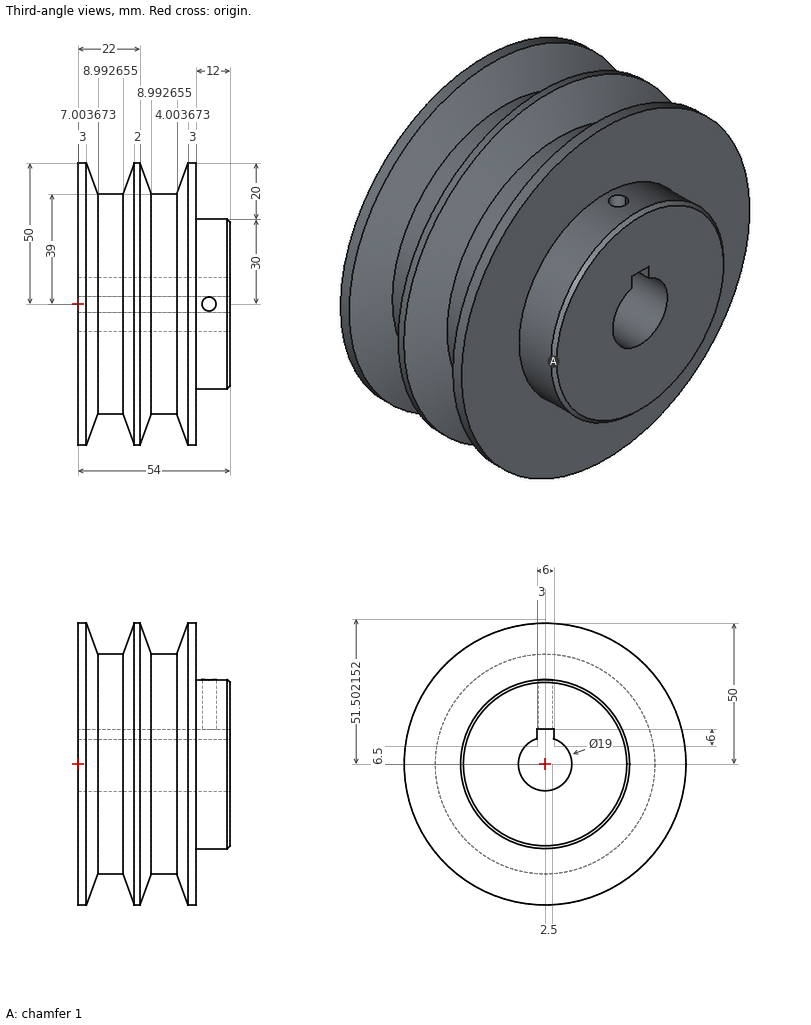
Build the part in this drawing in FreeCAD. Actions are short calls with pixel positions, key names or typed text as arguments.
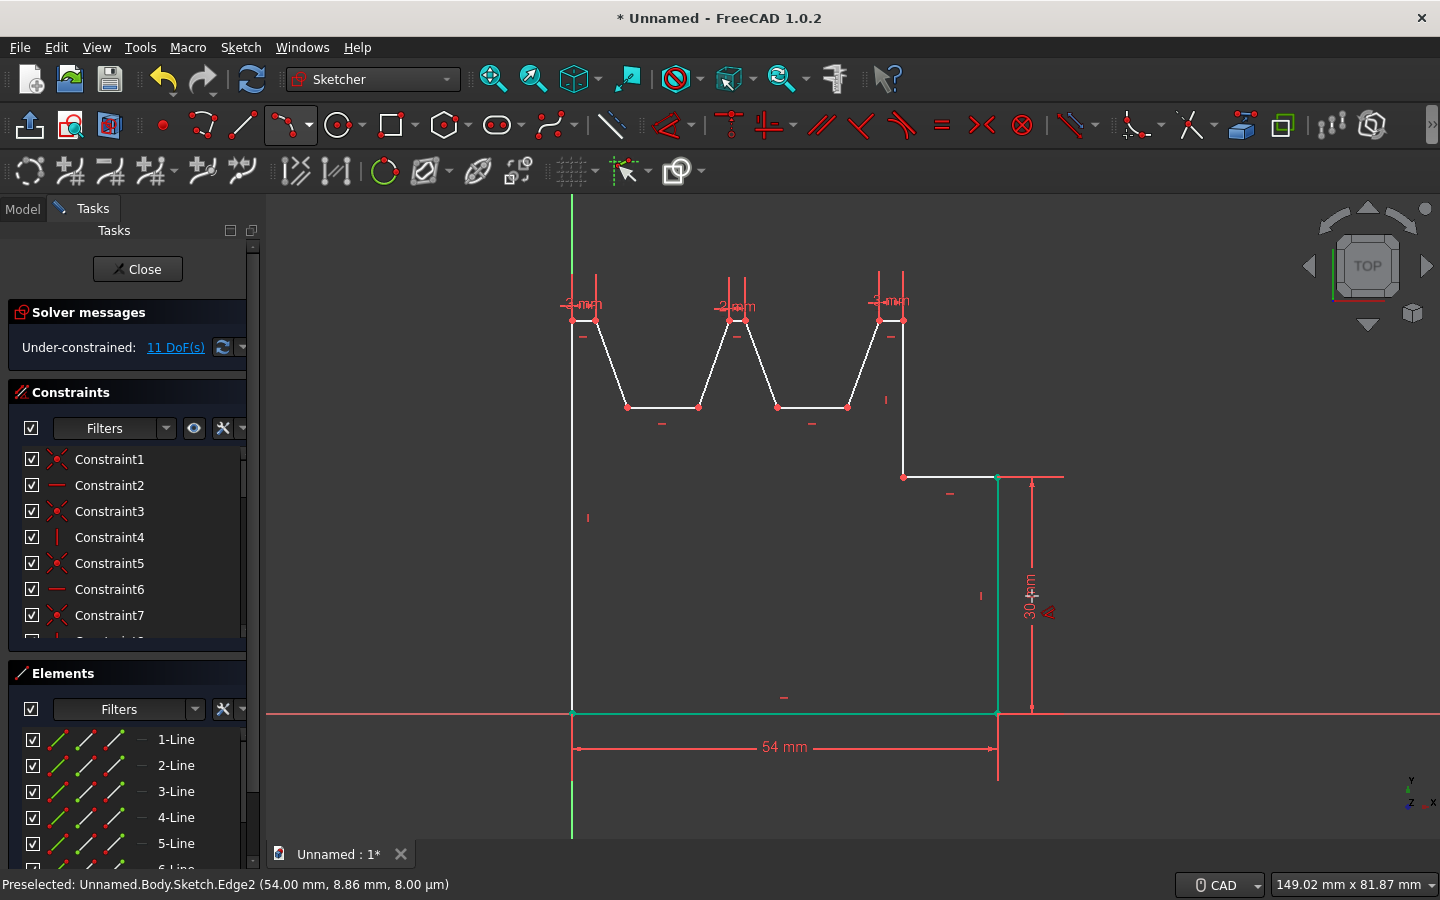
click(969, 477)
click(950, 443)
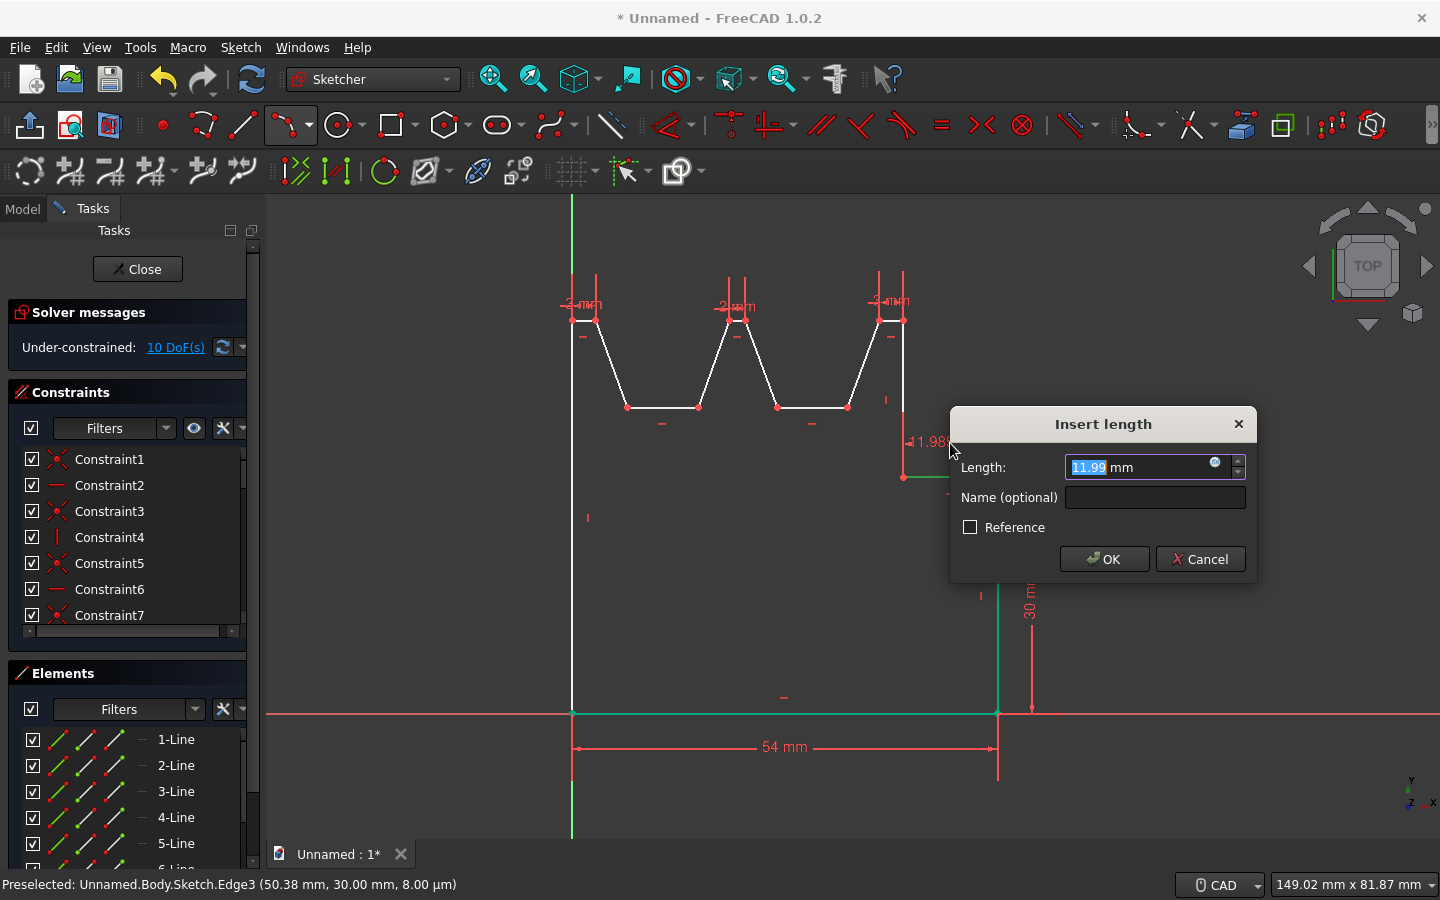
text(12)
key(Return)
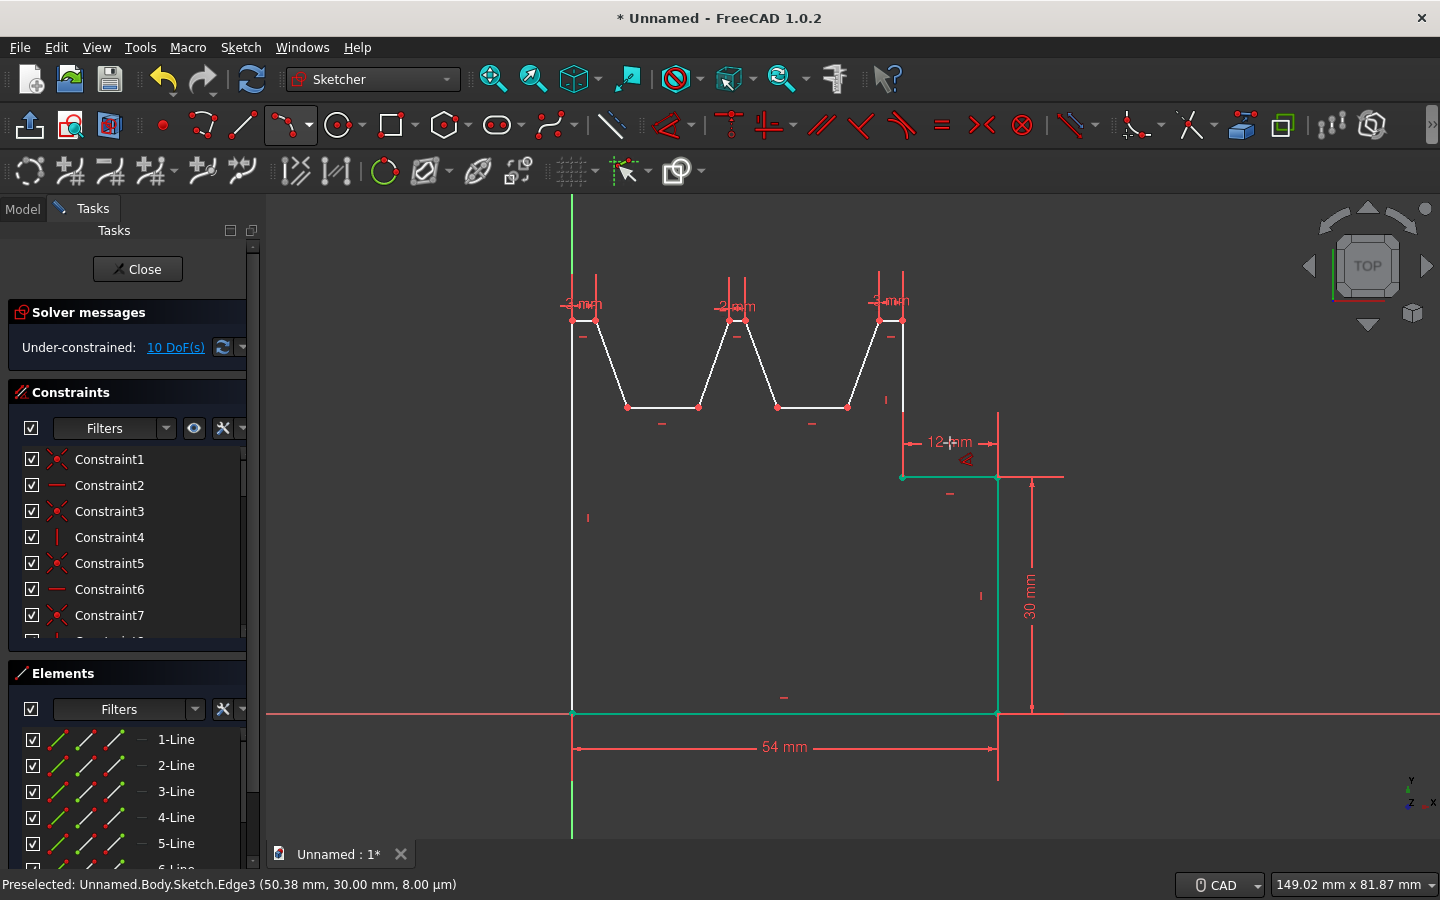
click(903, 430)
click(937, 399)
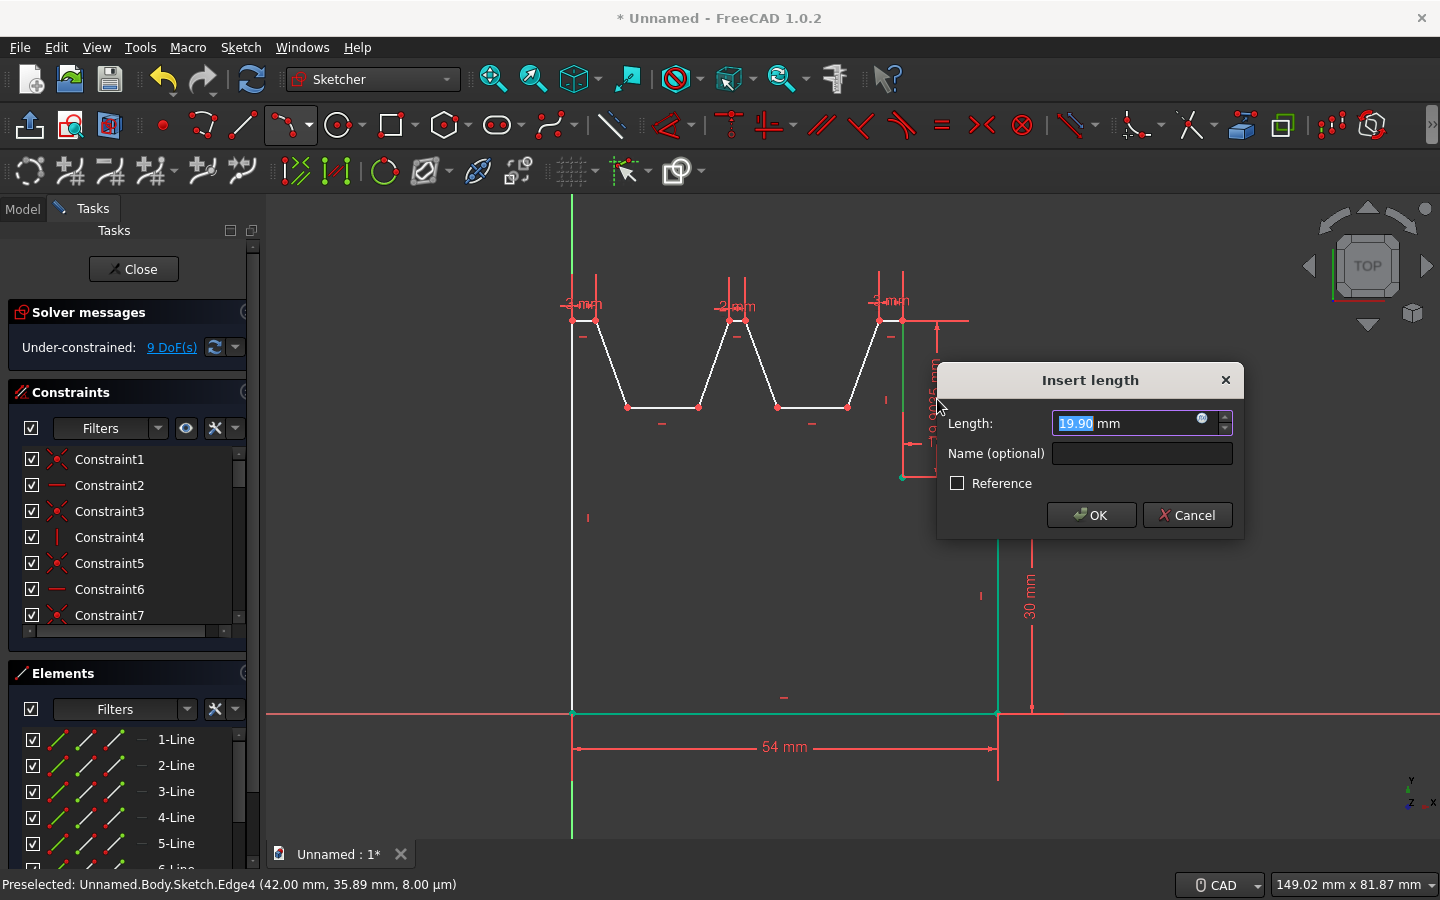
text(20)
key(Return)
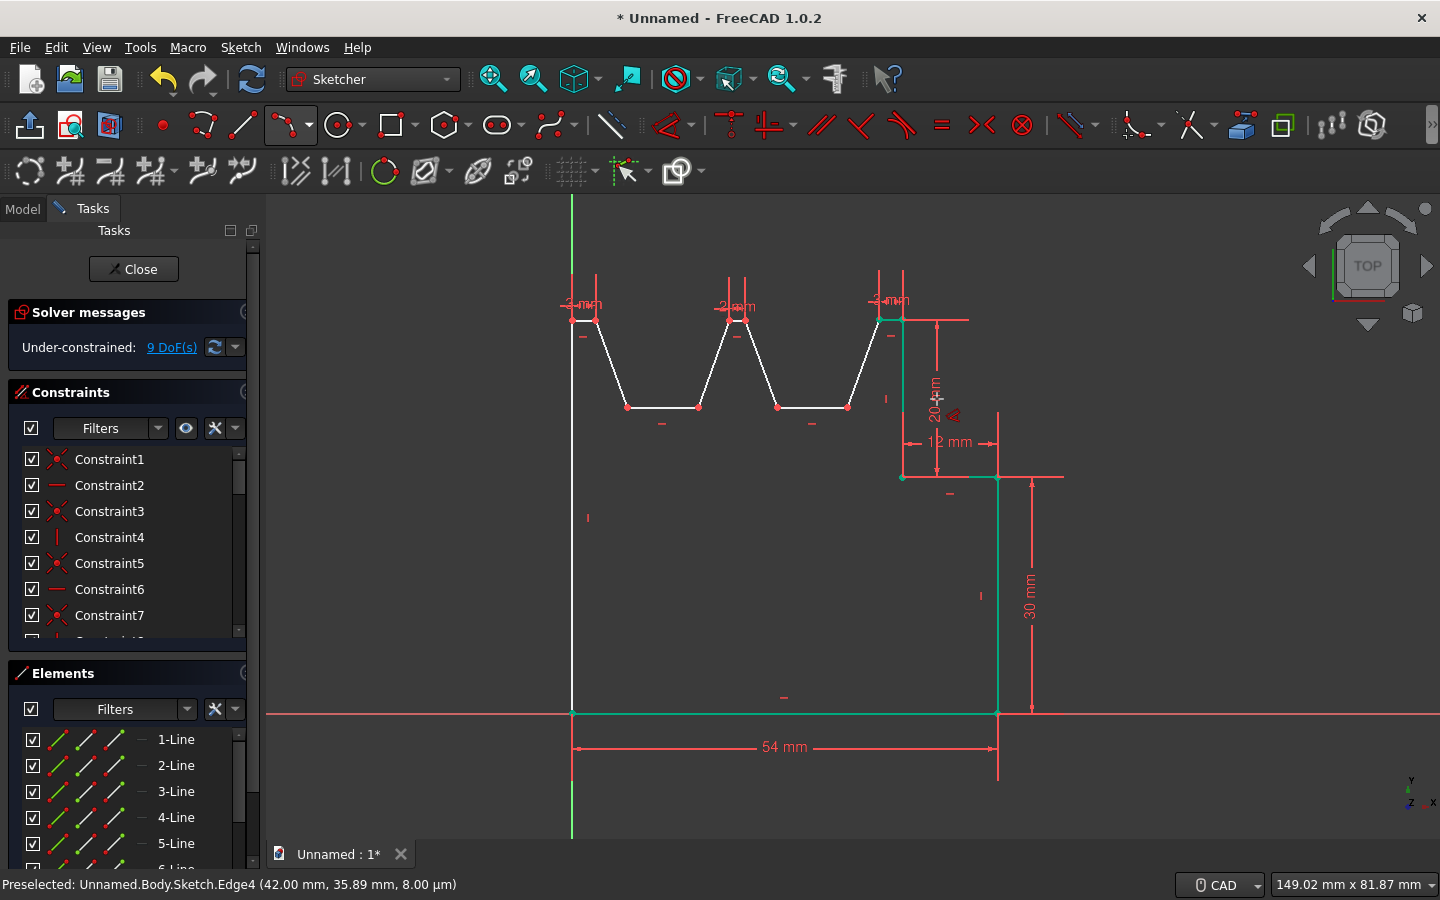
click(572, 439)
click(538, 517)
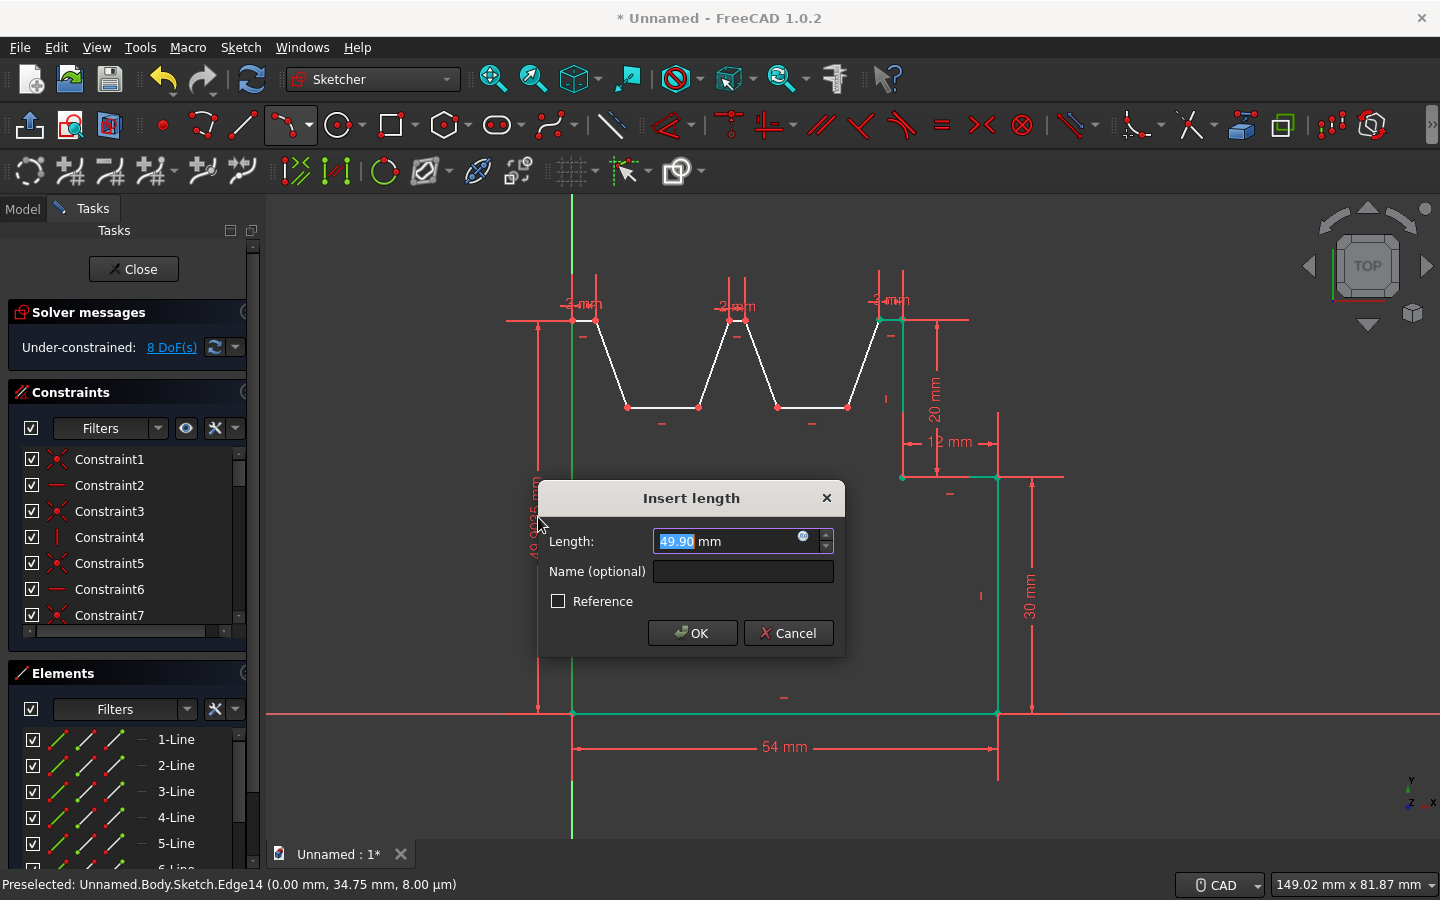
text(50)
key(Return)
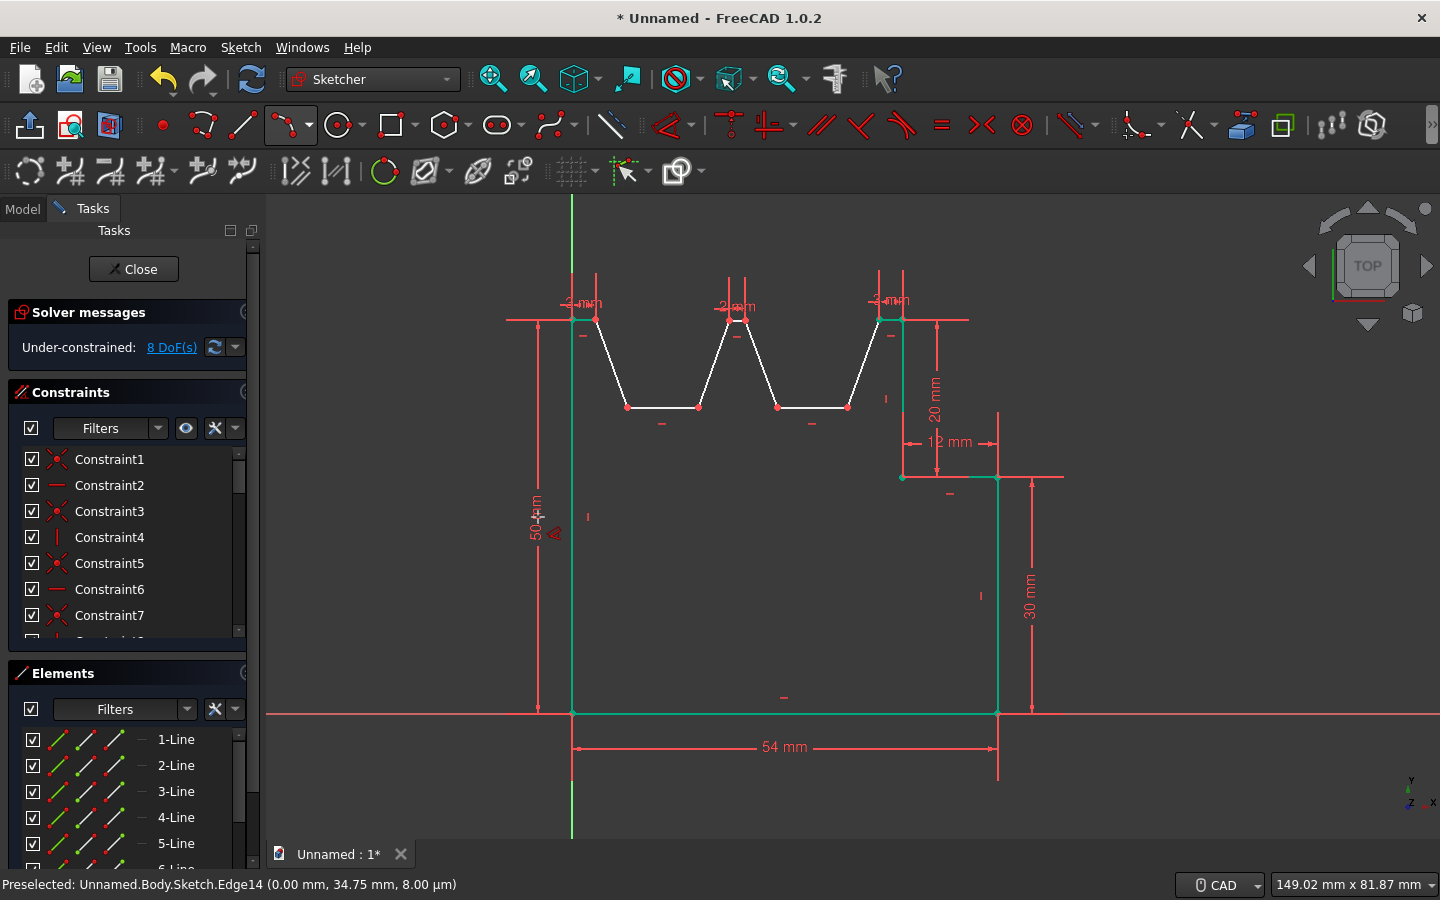
click(847, 408)
click(538, 561)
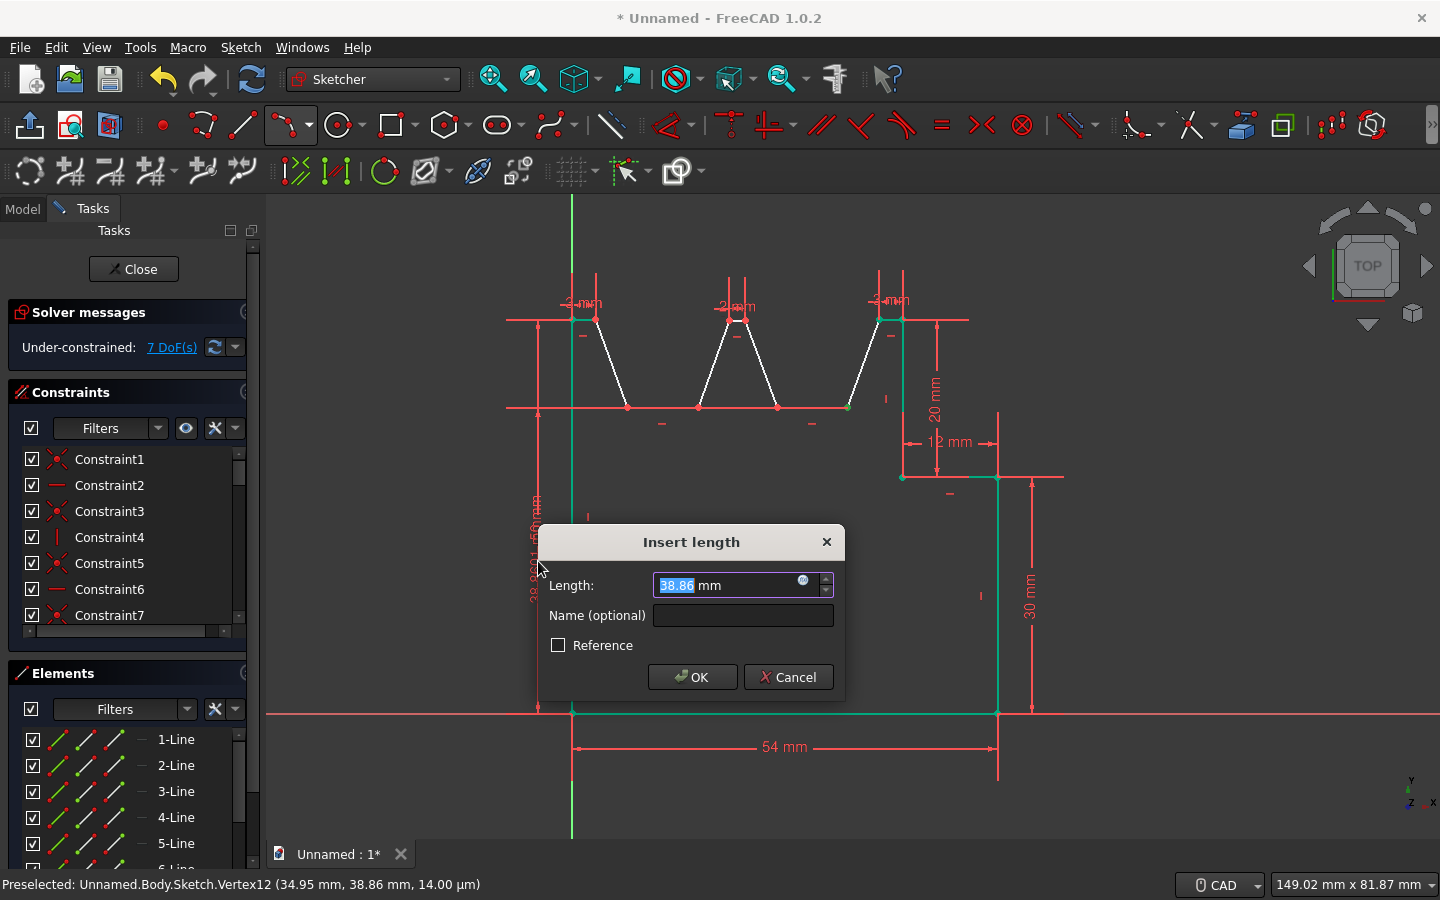
text(39)
key(Return)